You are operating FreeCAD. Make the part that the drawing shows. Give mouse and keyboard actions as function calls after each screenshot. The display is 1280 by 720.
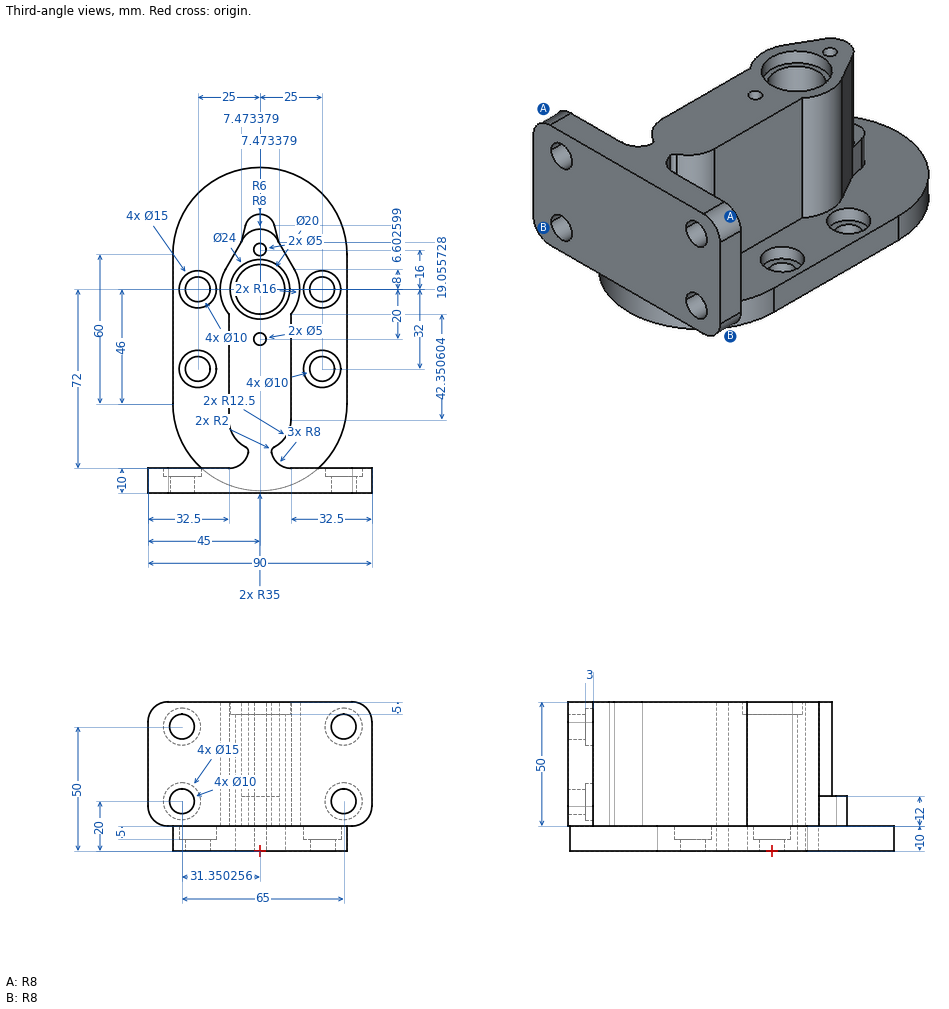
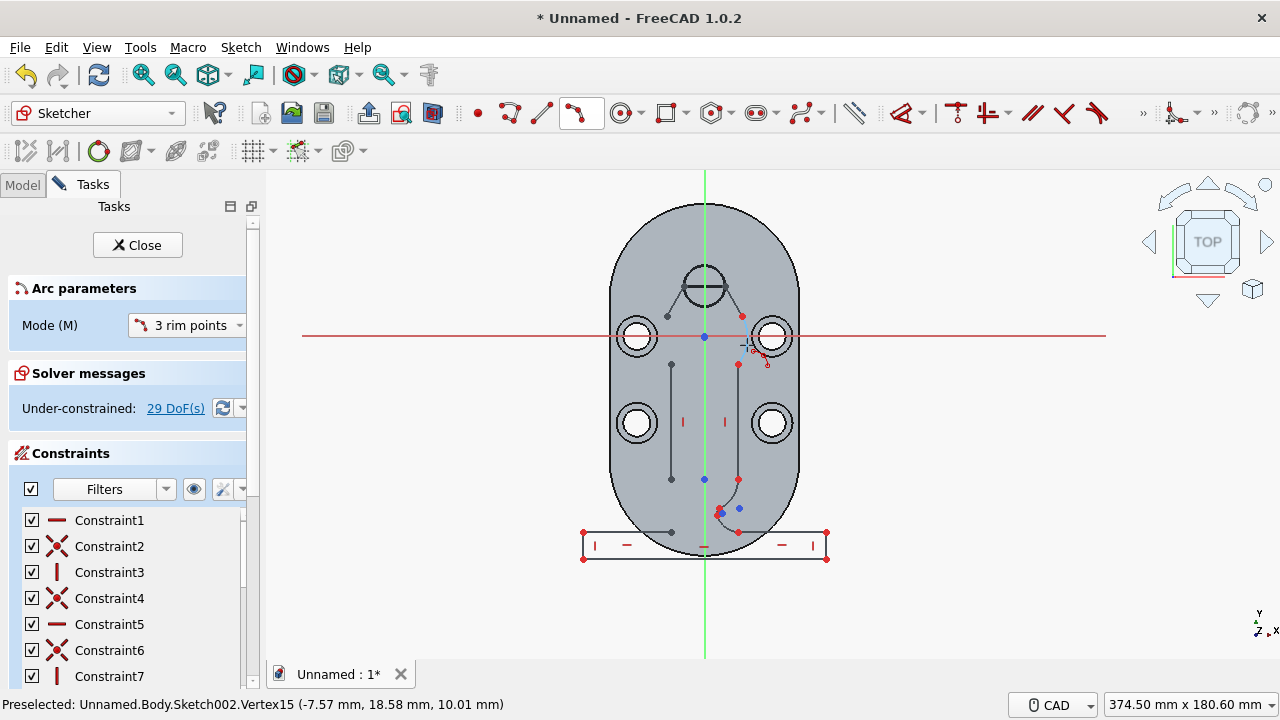
scroll(694, 273, up, 3)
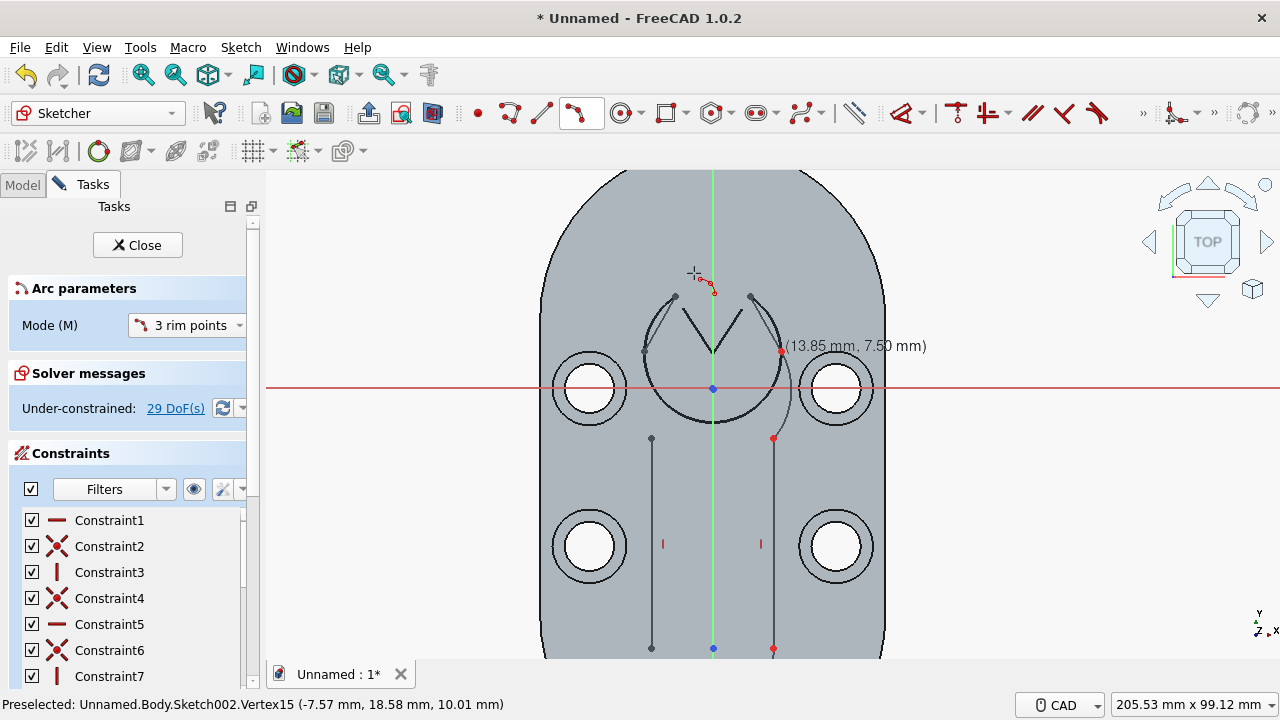
click(694, 274)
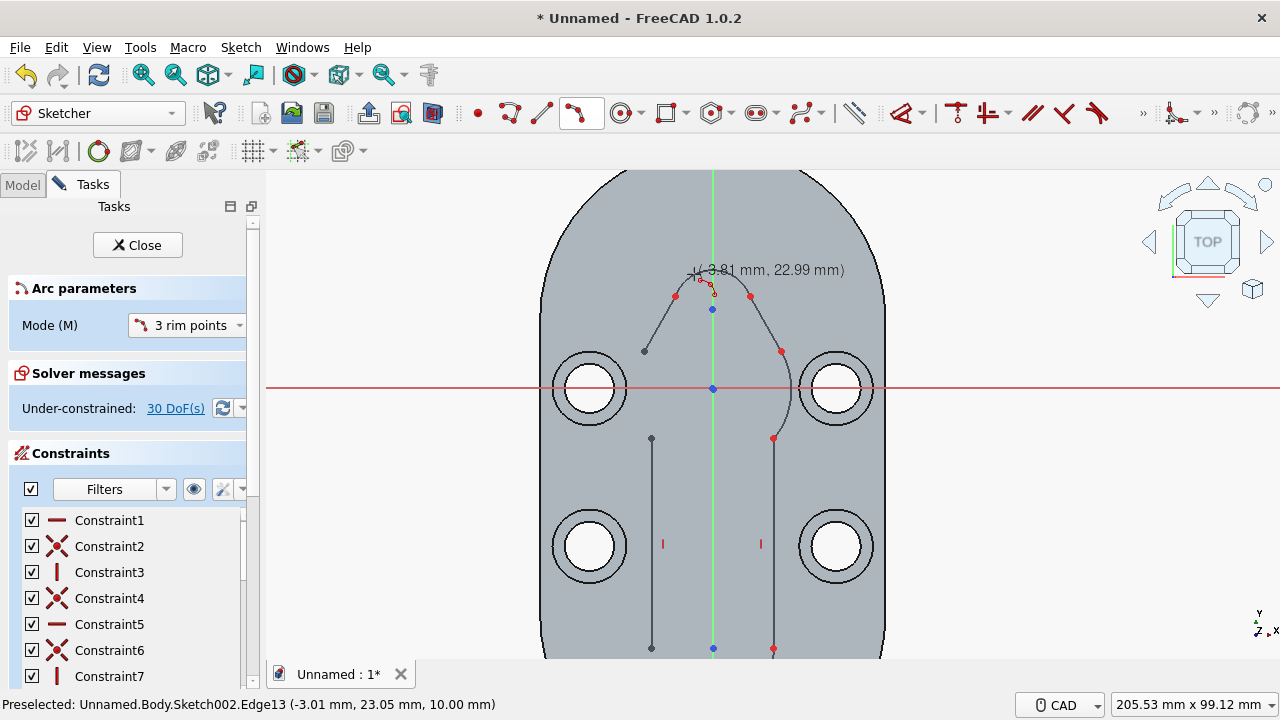
click(644, 351)
click(652, 439)
click(635, 404)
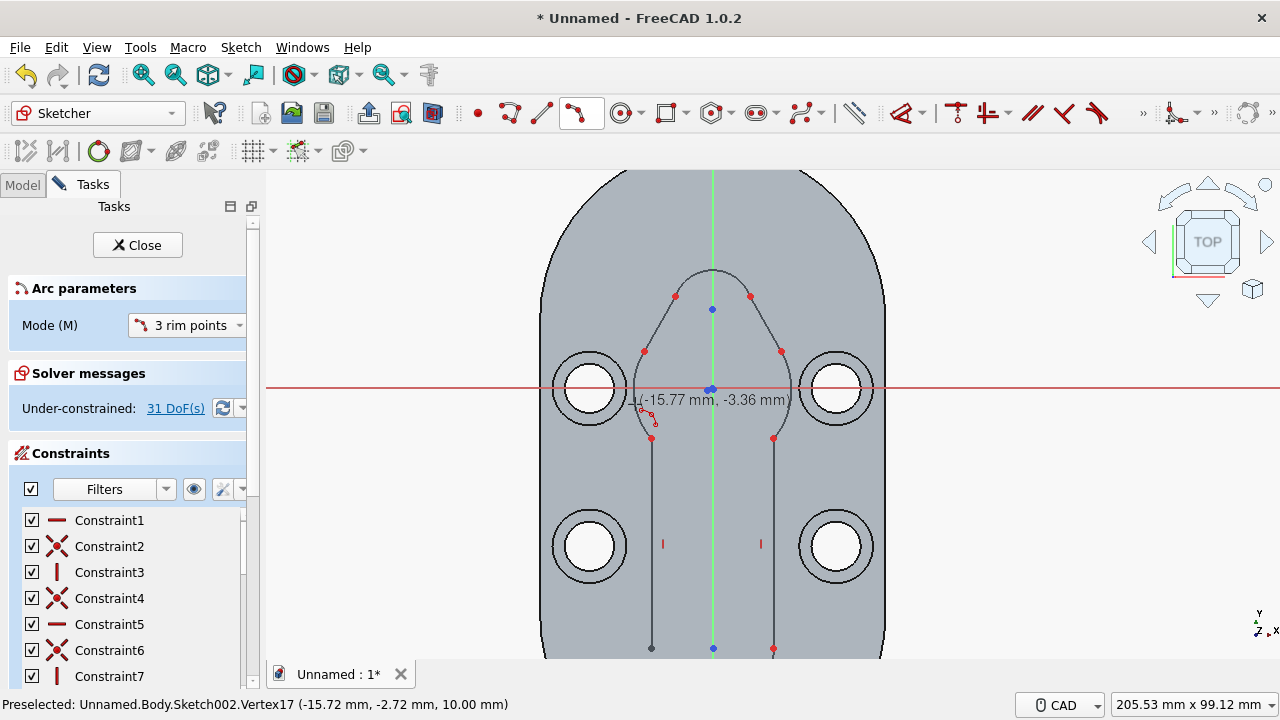
scroll(694, 273, down, 3)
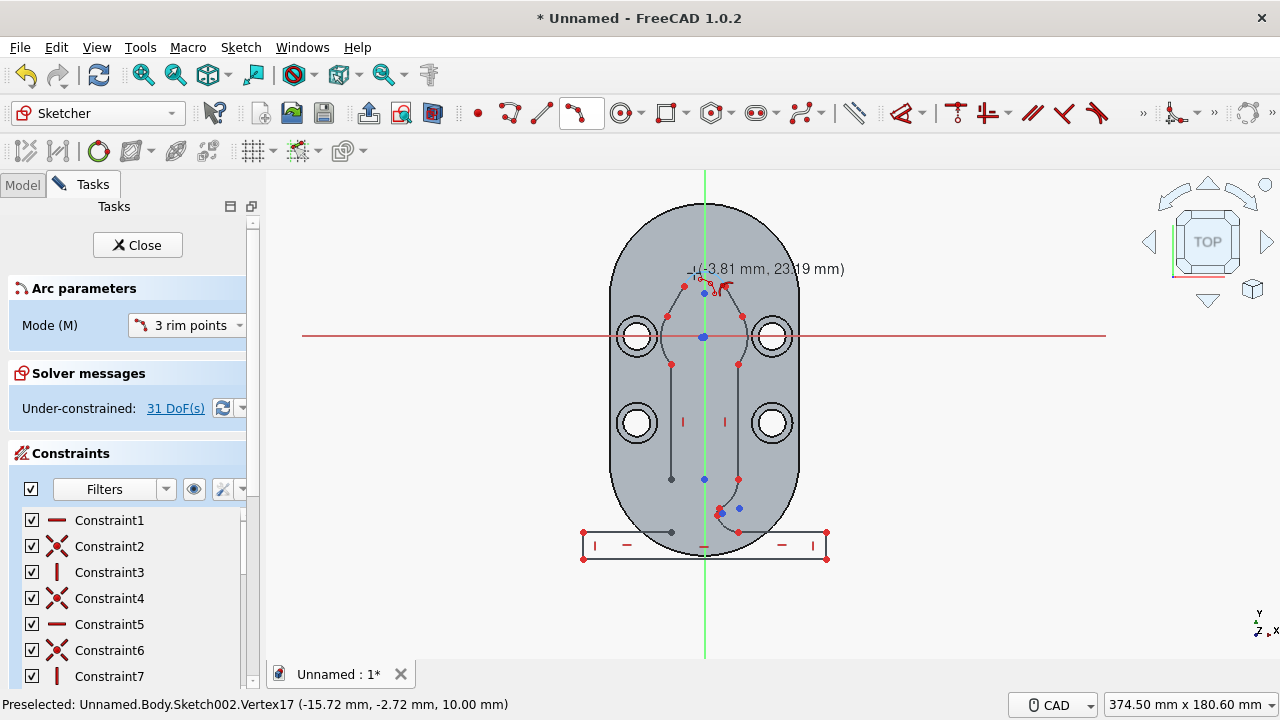
click(671, 479)
click(689, 508)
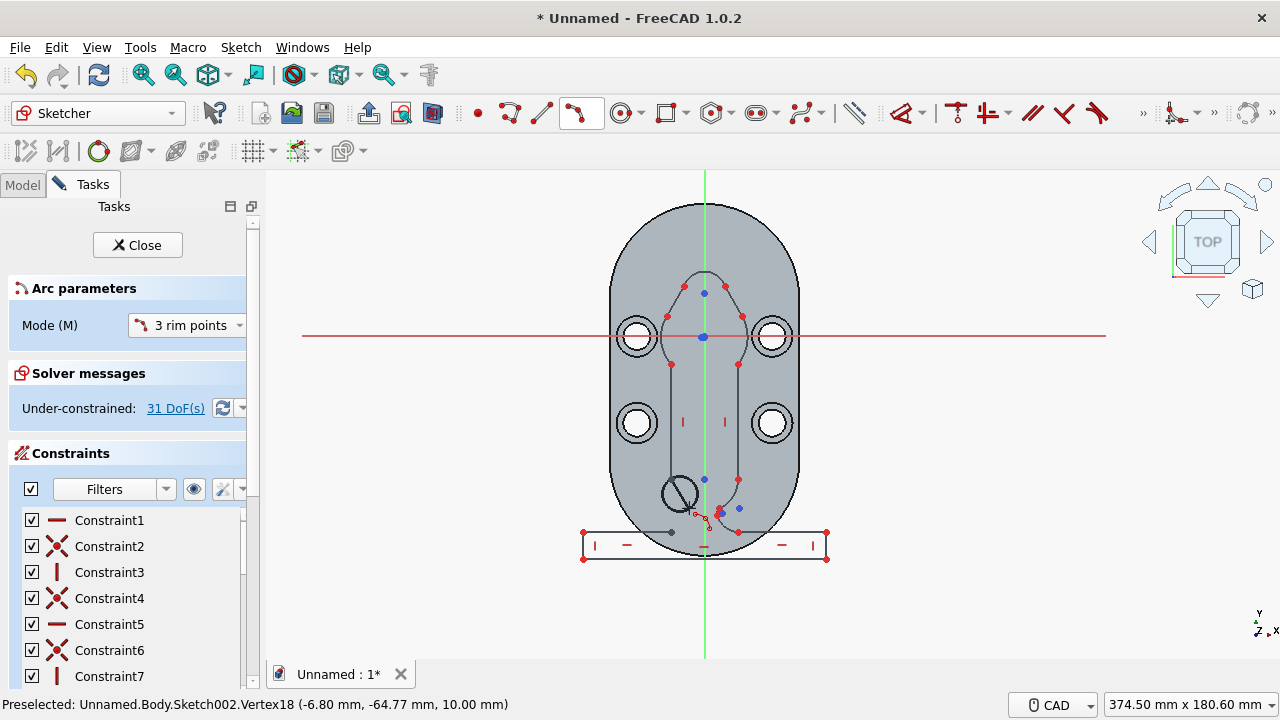
scroll(676, 496, up, 6)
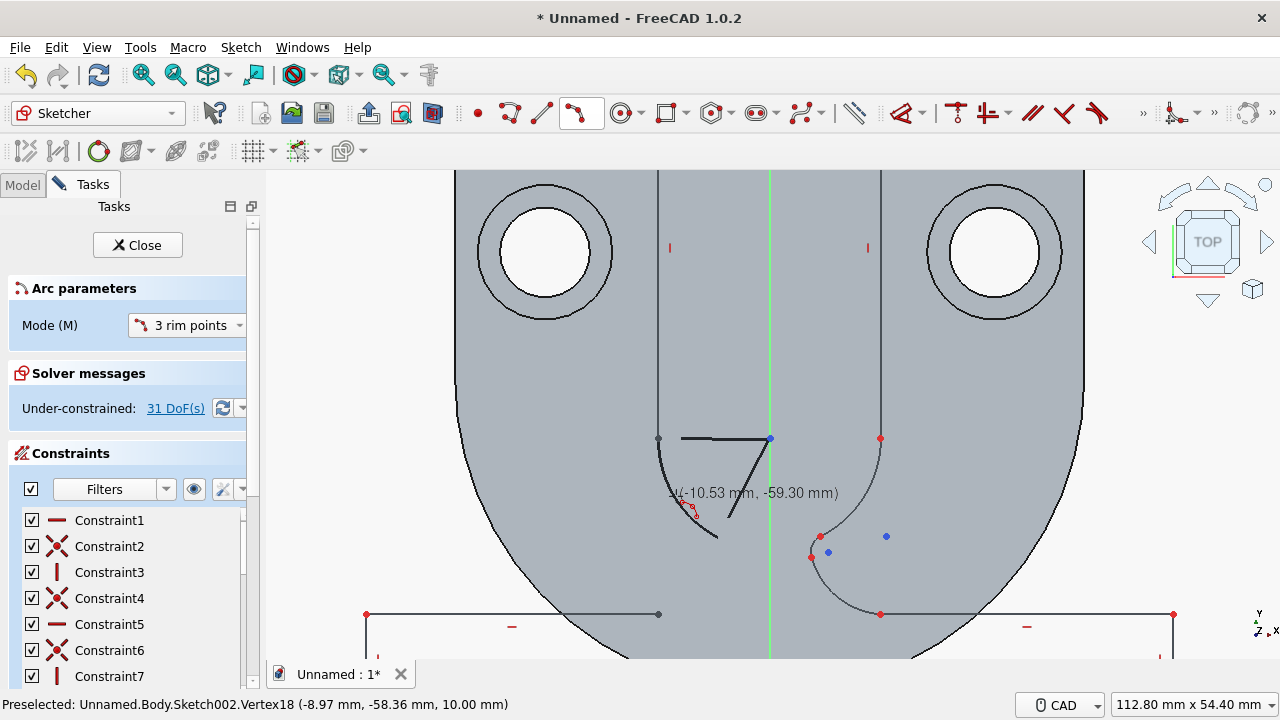
click(674, 494)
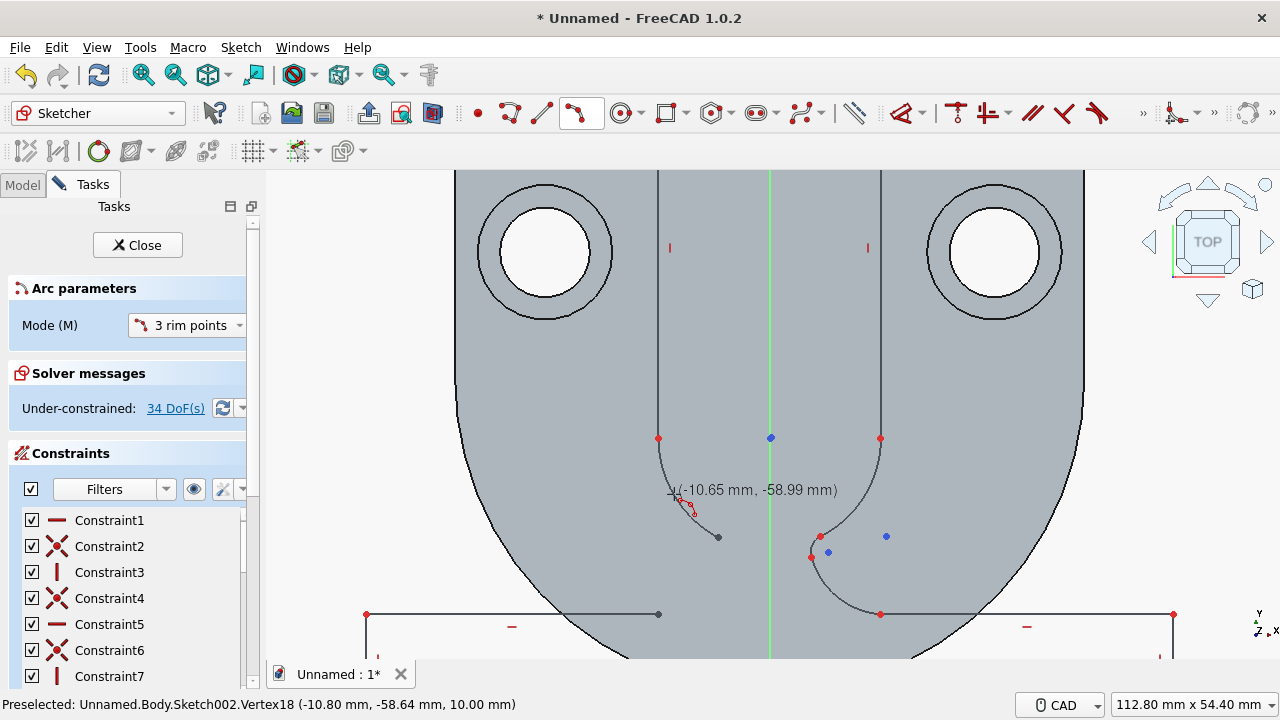
click(718, 538)
click(728, 555)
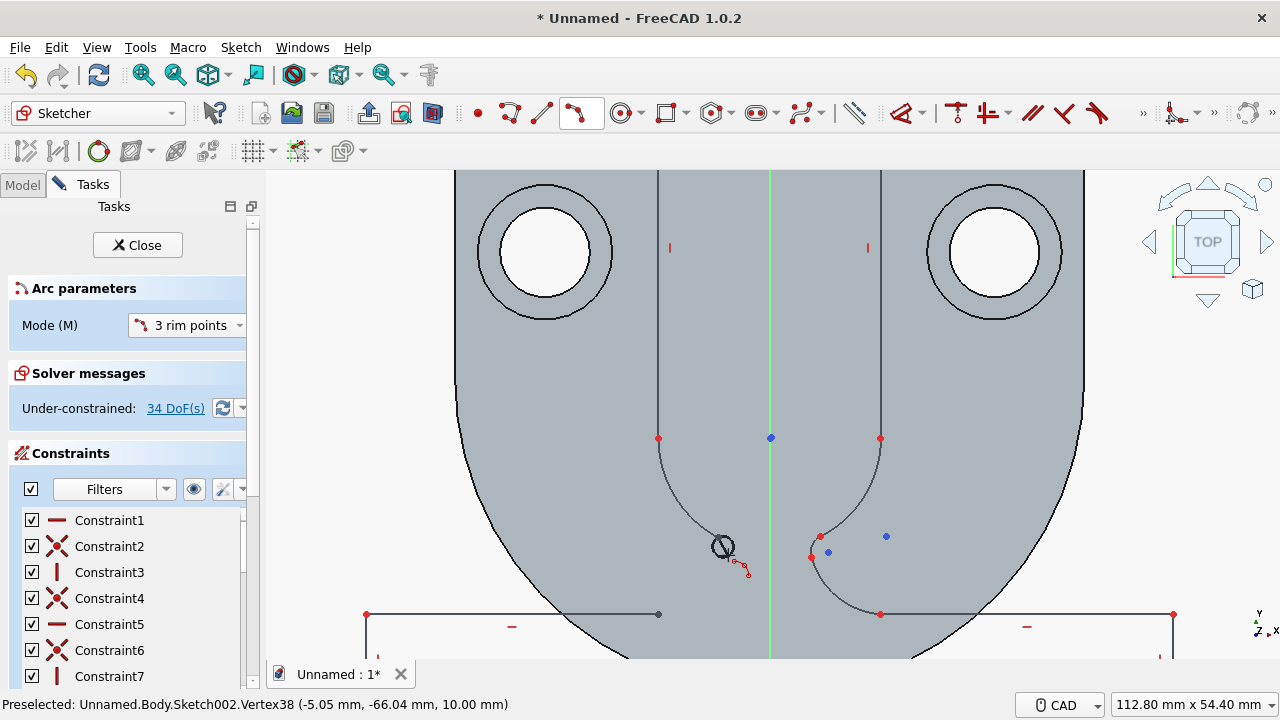
scroll(726, 543, up, 8)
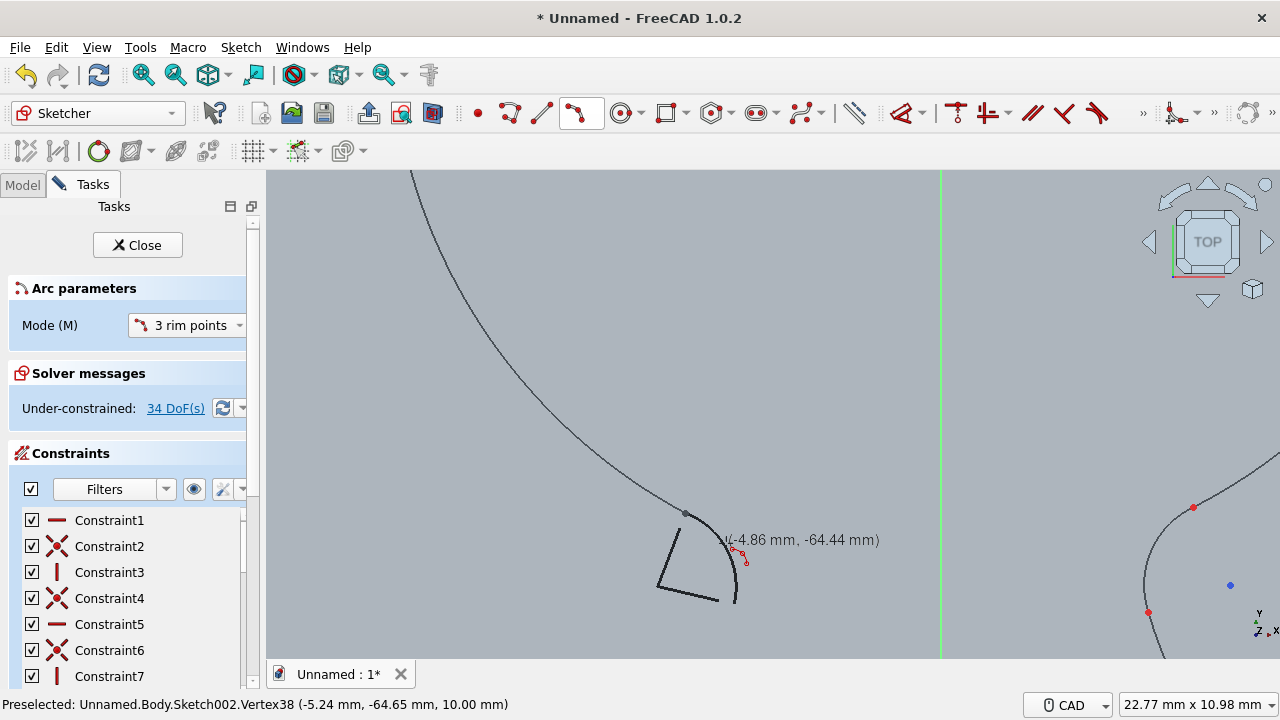
click(726, 542)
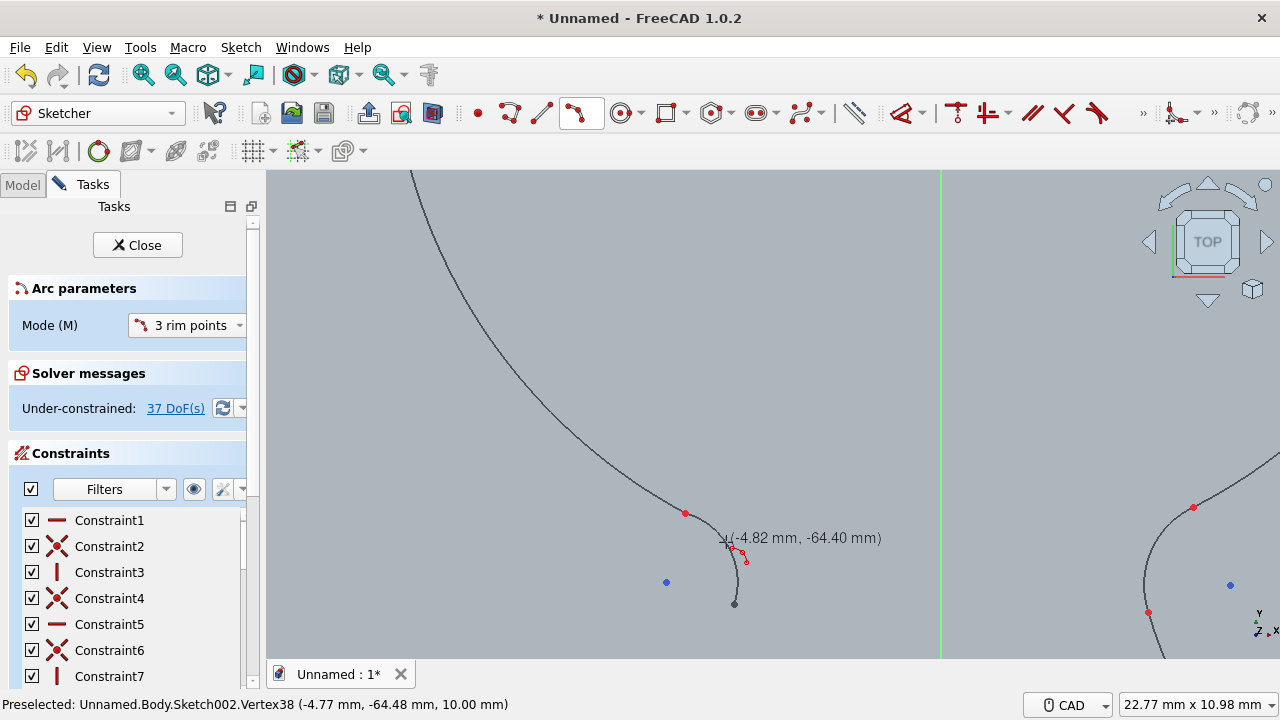
scroll(689, 509, down, 14)